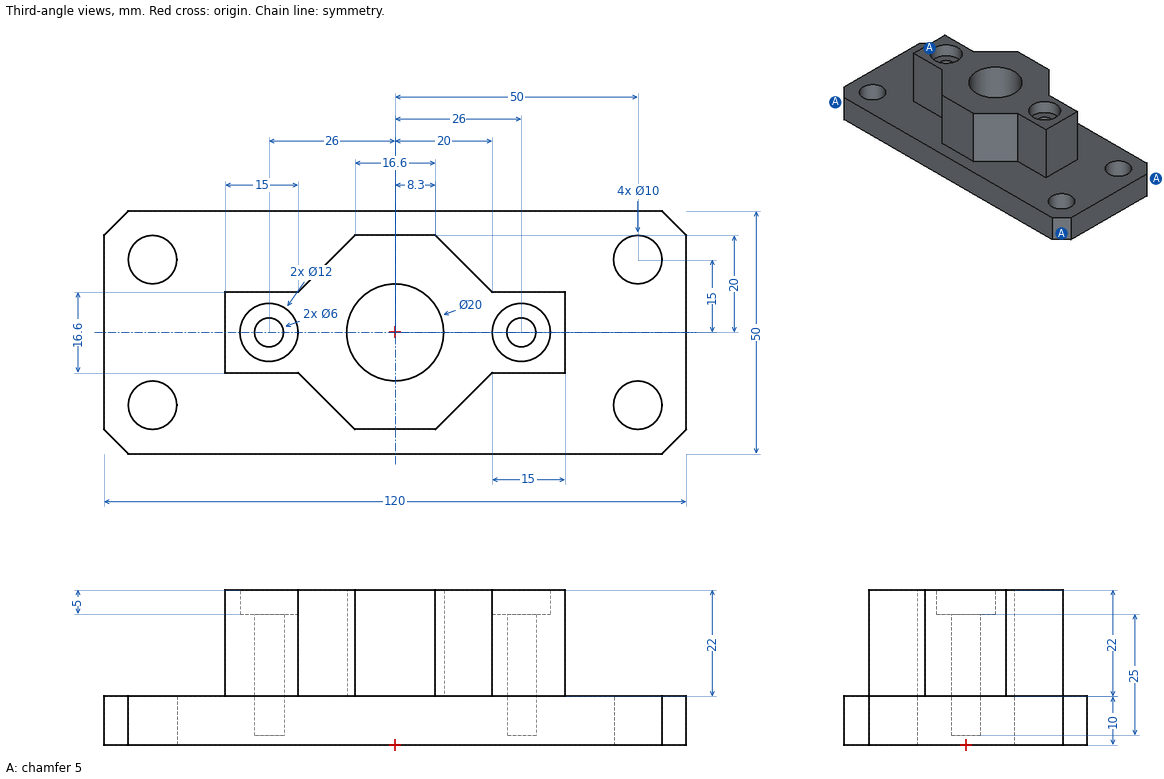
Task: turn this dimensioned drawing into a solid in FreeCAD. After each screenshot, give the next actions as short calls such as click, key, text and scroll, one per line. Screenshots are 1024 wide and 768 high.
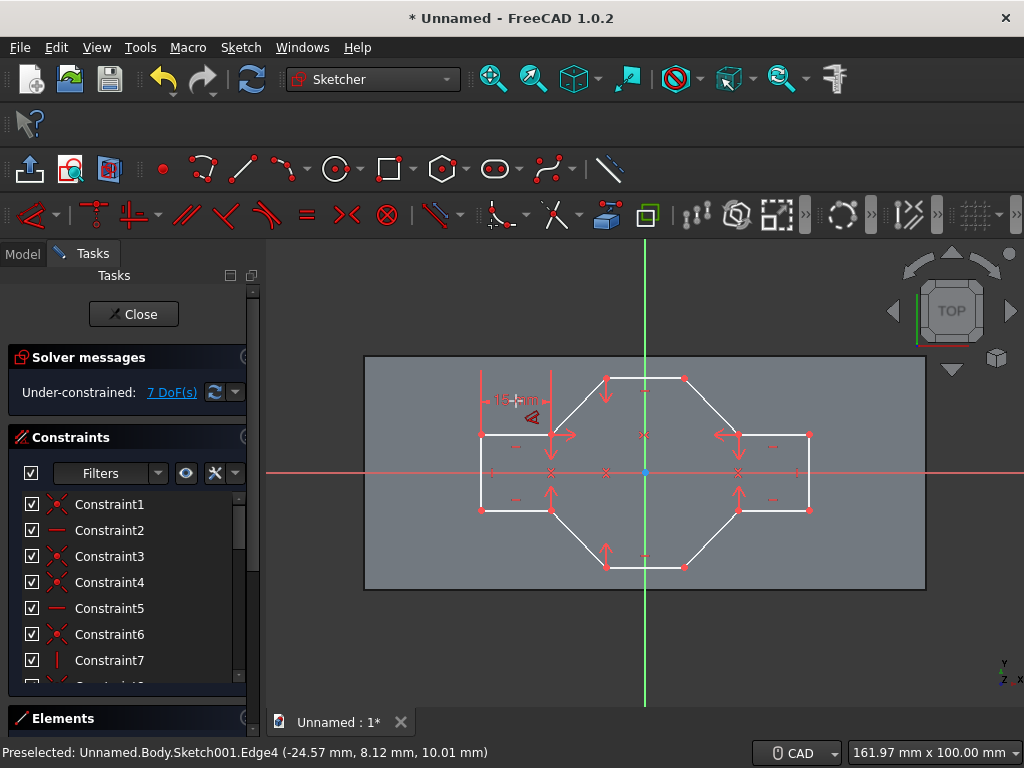
click(760, 511)
click(774, 545)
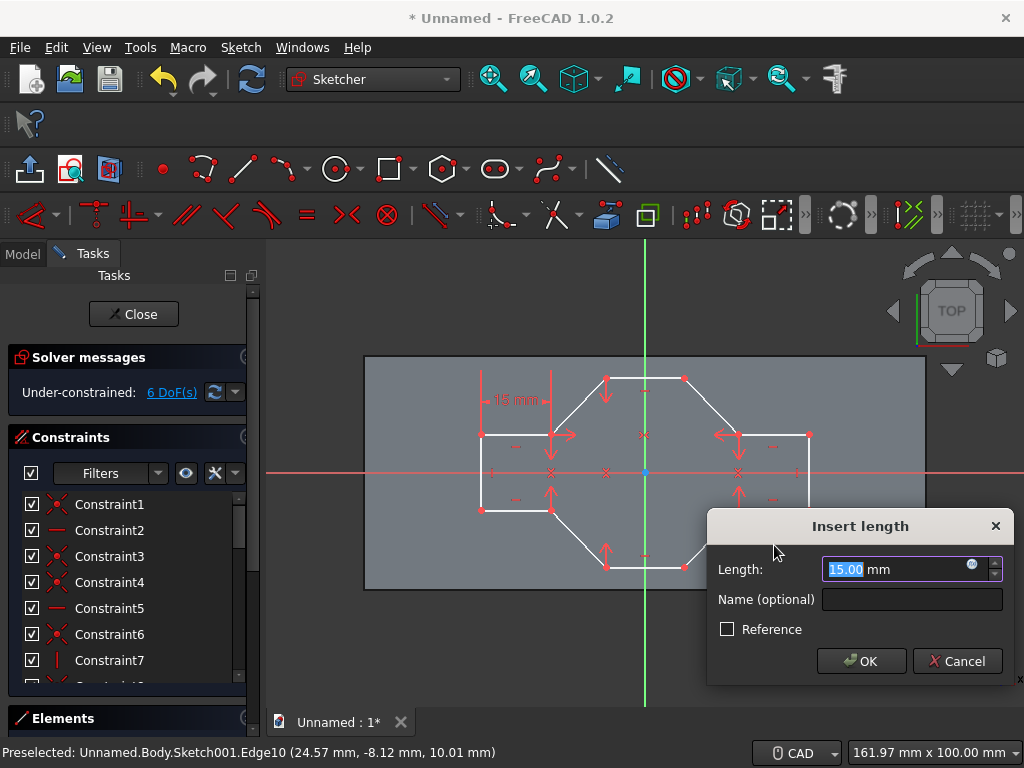
text(15)
key(Return)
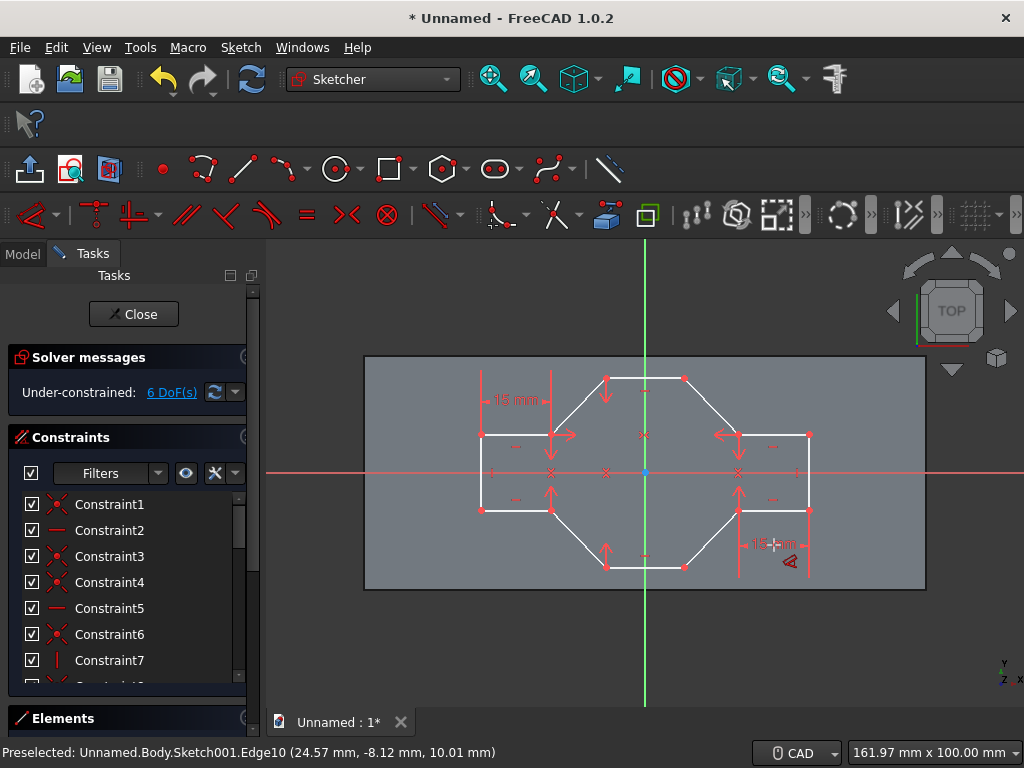
click(739, 435)
click(670, 401)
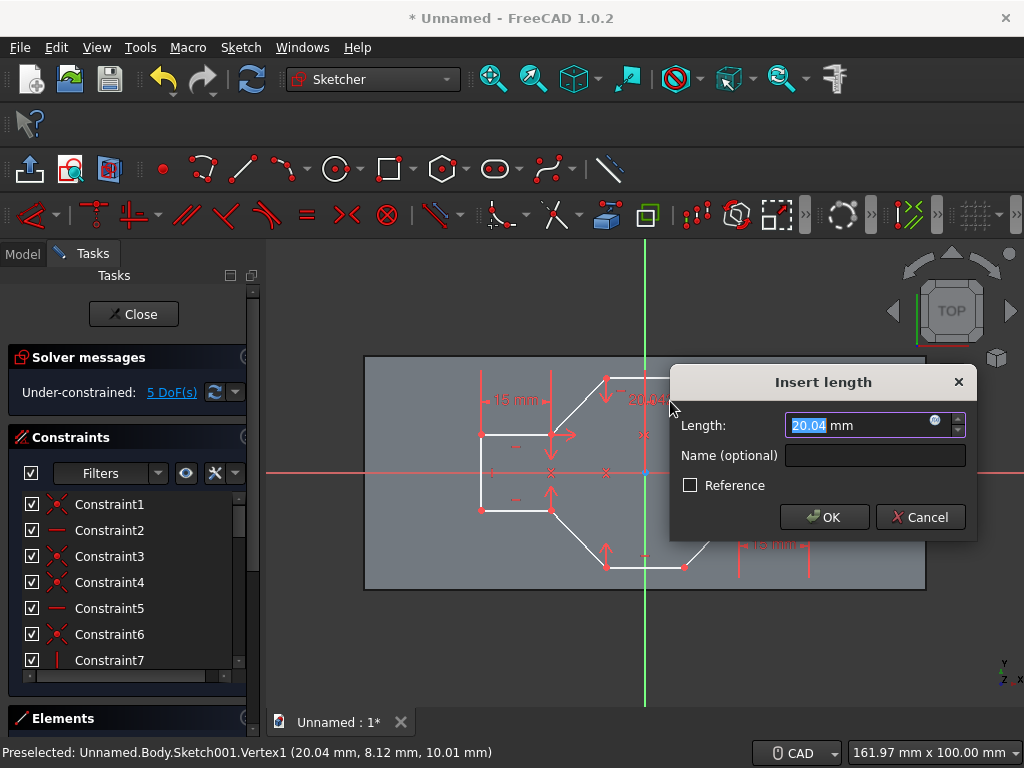
text(20)
key(Return)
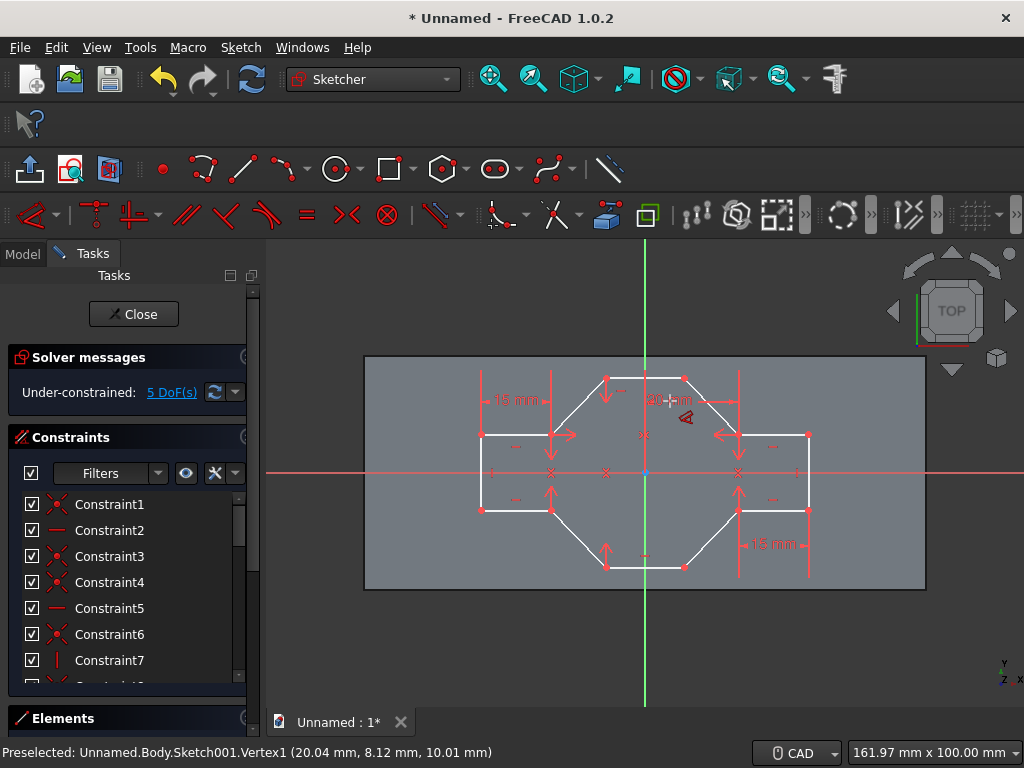
click(684, 378)
click(718, 447)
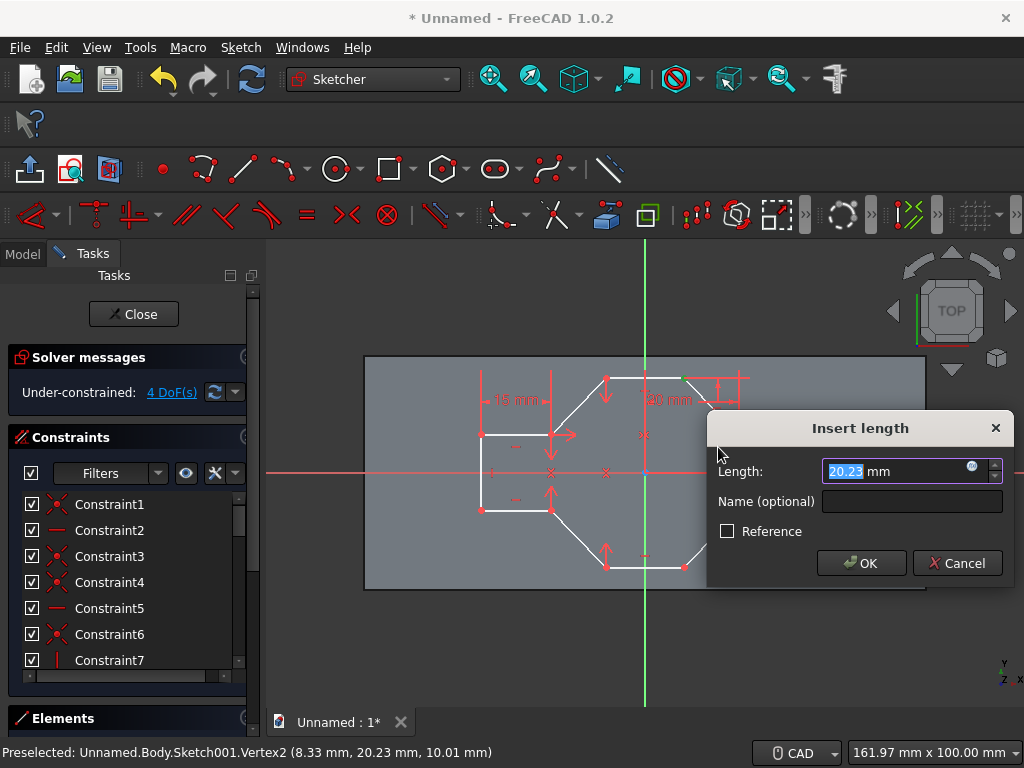
text(20)
key(Return)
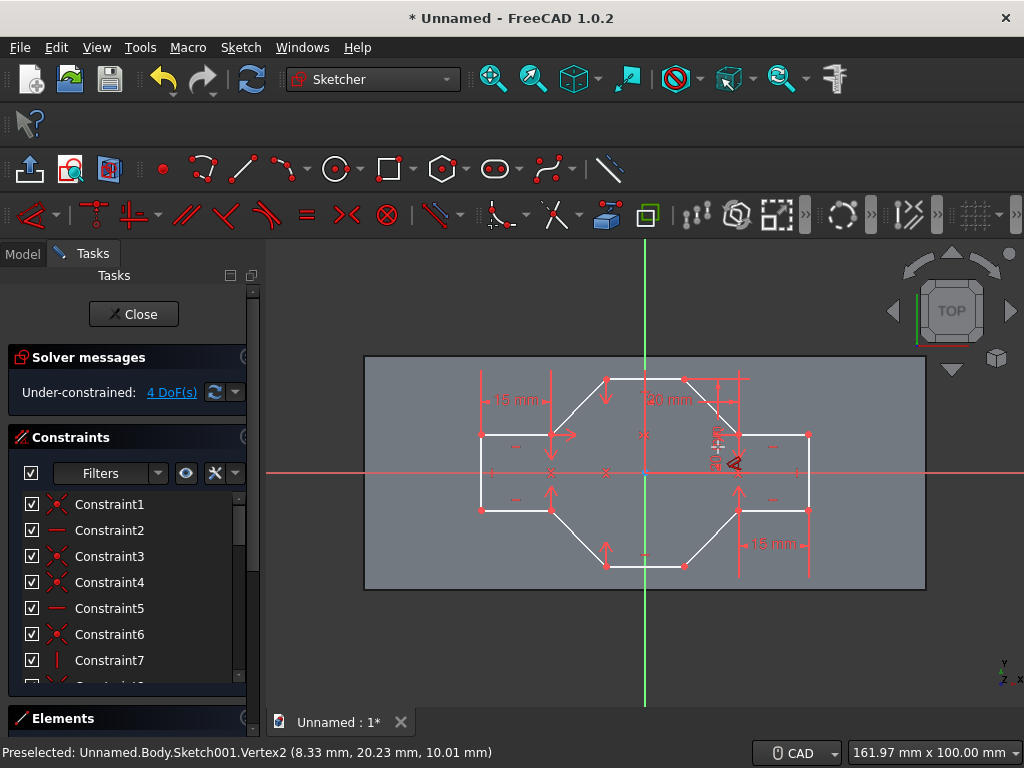
click(661, 379)
click(627, 345)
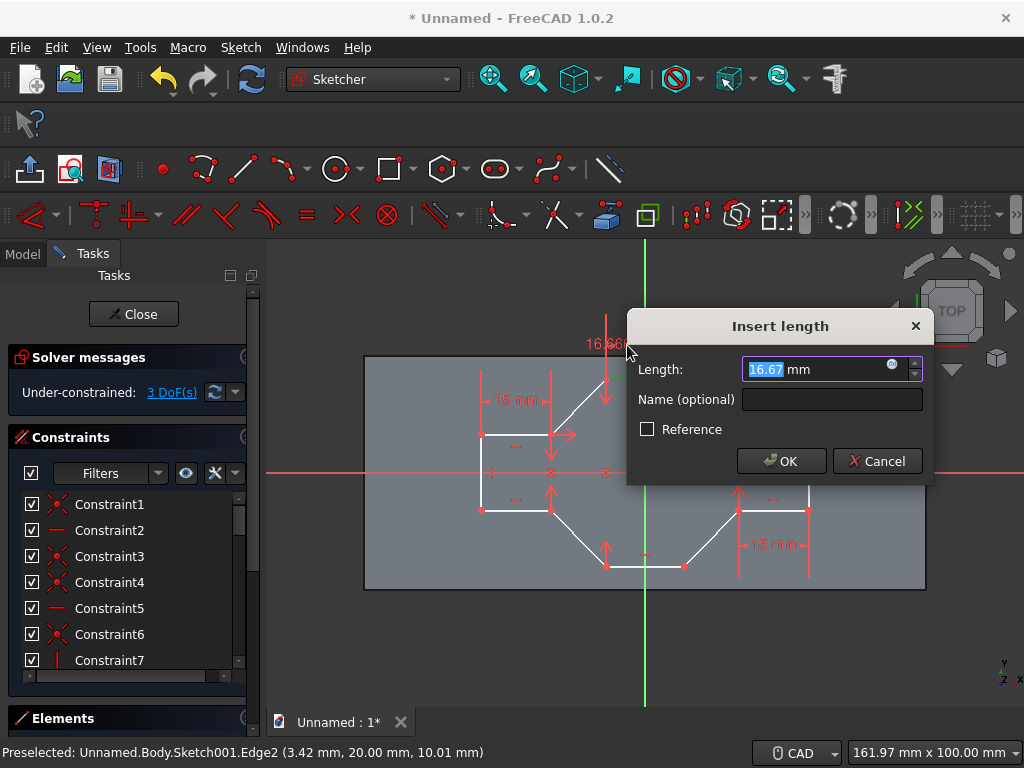
text(16.6)
key(Return)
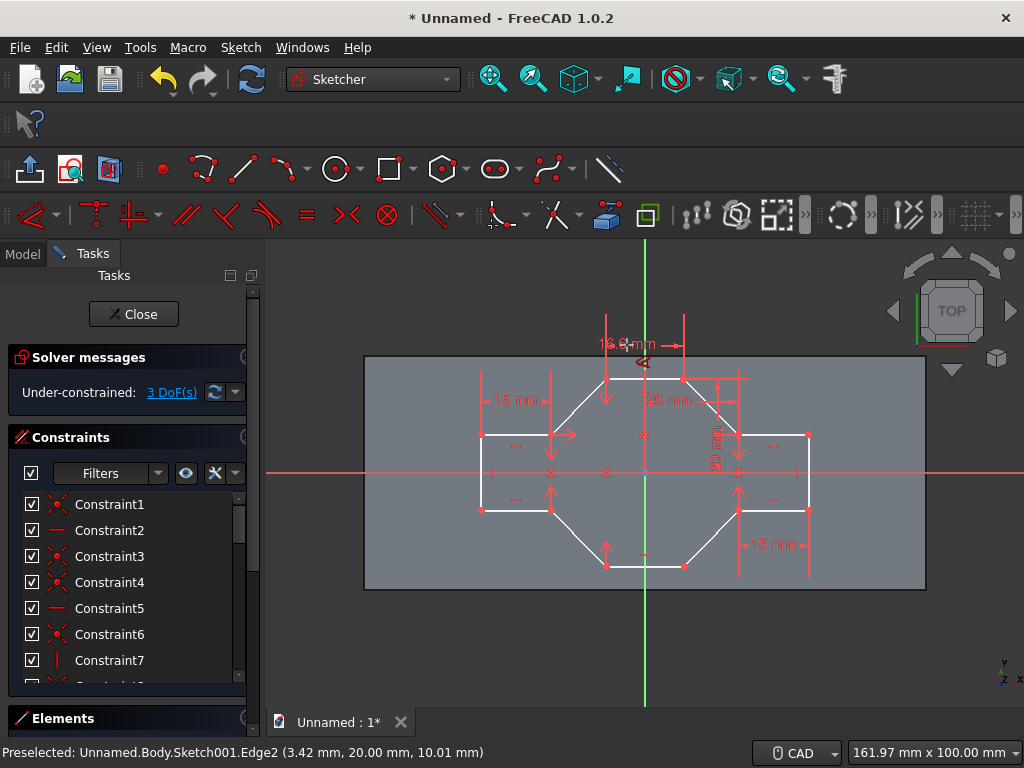
click(481, 458)
click(447, 456)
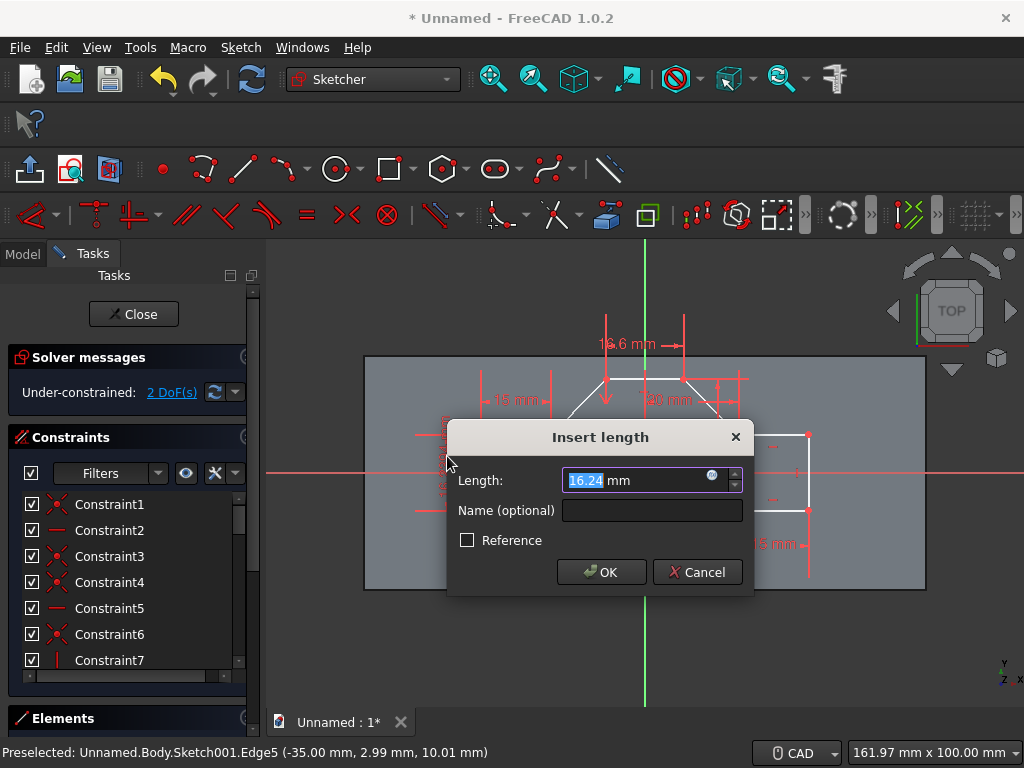
text(16.6)
key(Return)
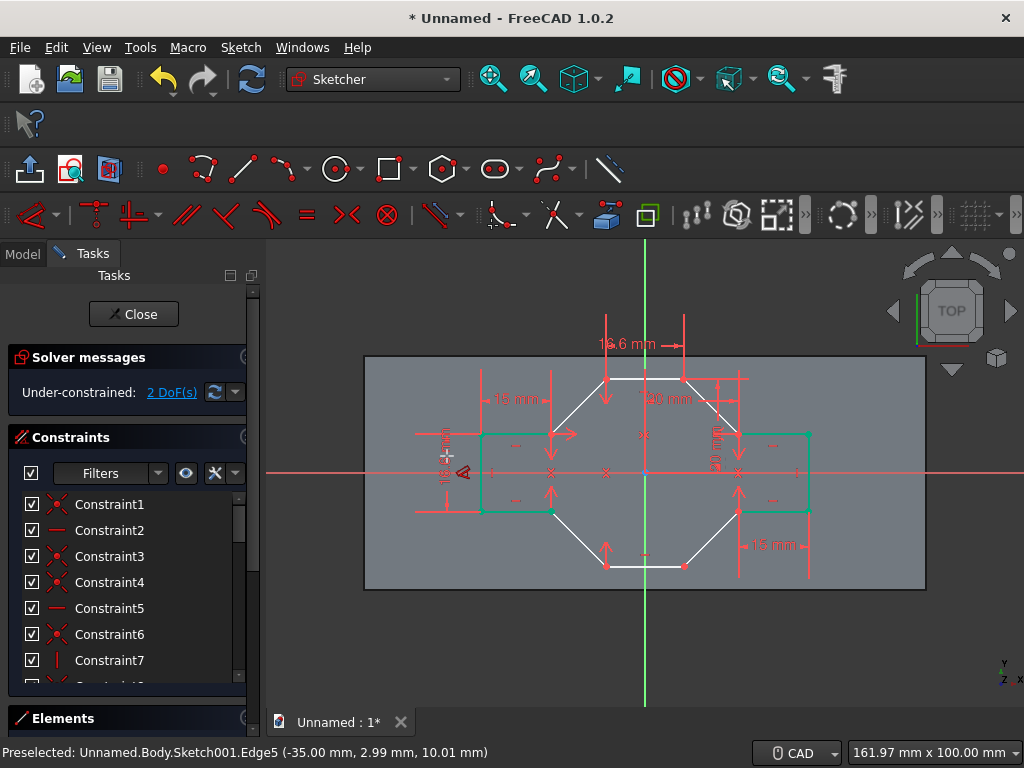
click(629, 567)
click(627, 601)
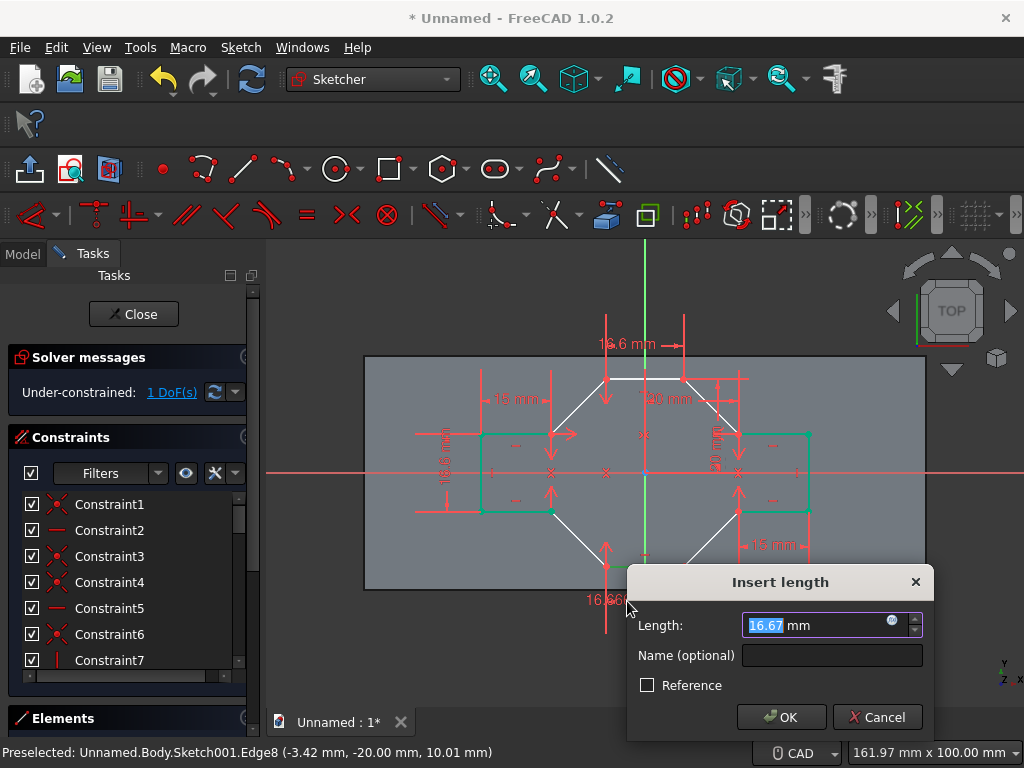
text(16.6)
key(Return)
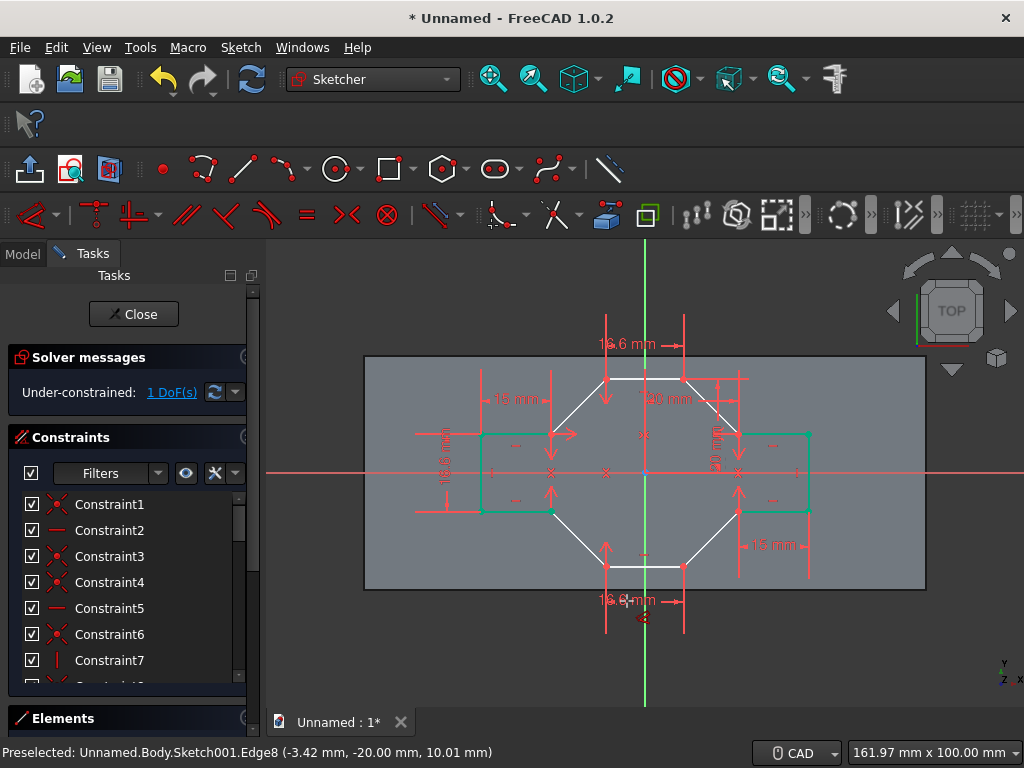
click(684, 379)
click(664, 507)